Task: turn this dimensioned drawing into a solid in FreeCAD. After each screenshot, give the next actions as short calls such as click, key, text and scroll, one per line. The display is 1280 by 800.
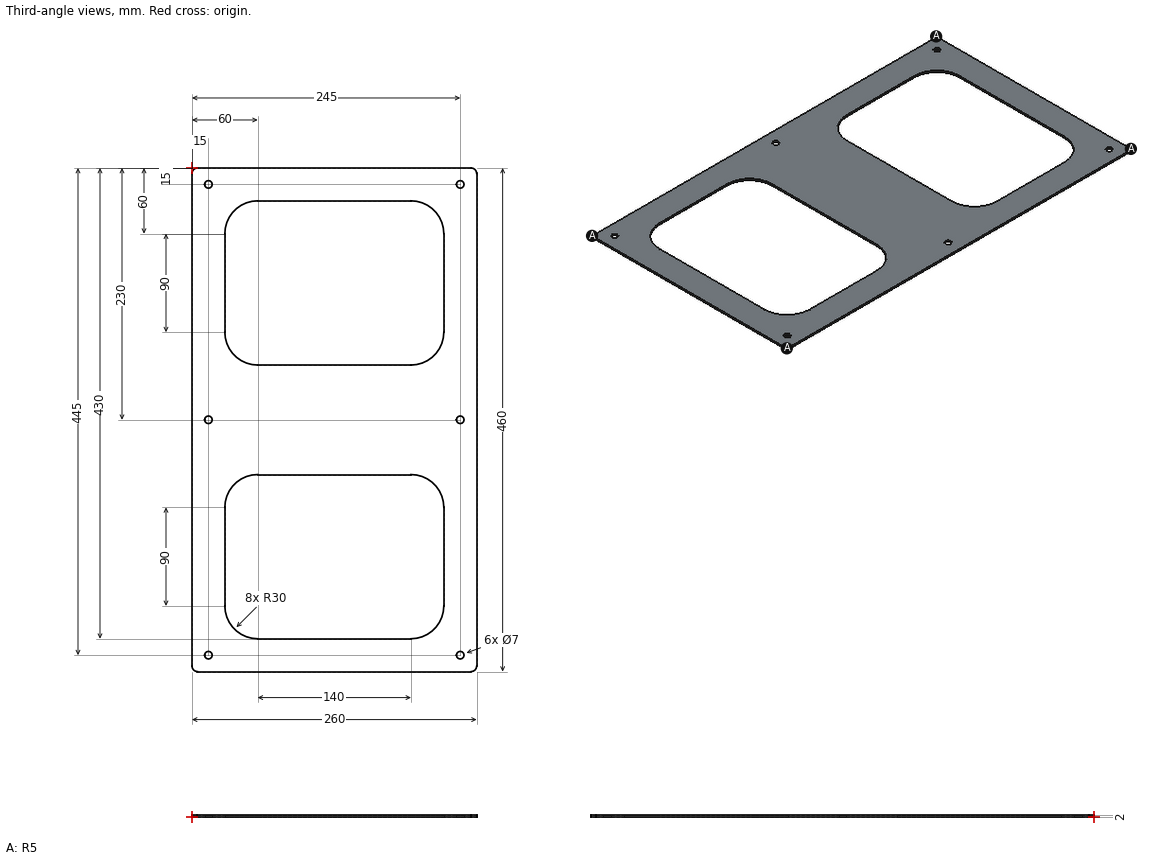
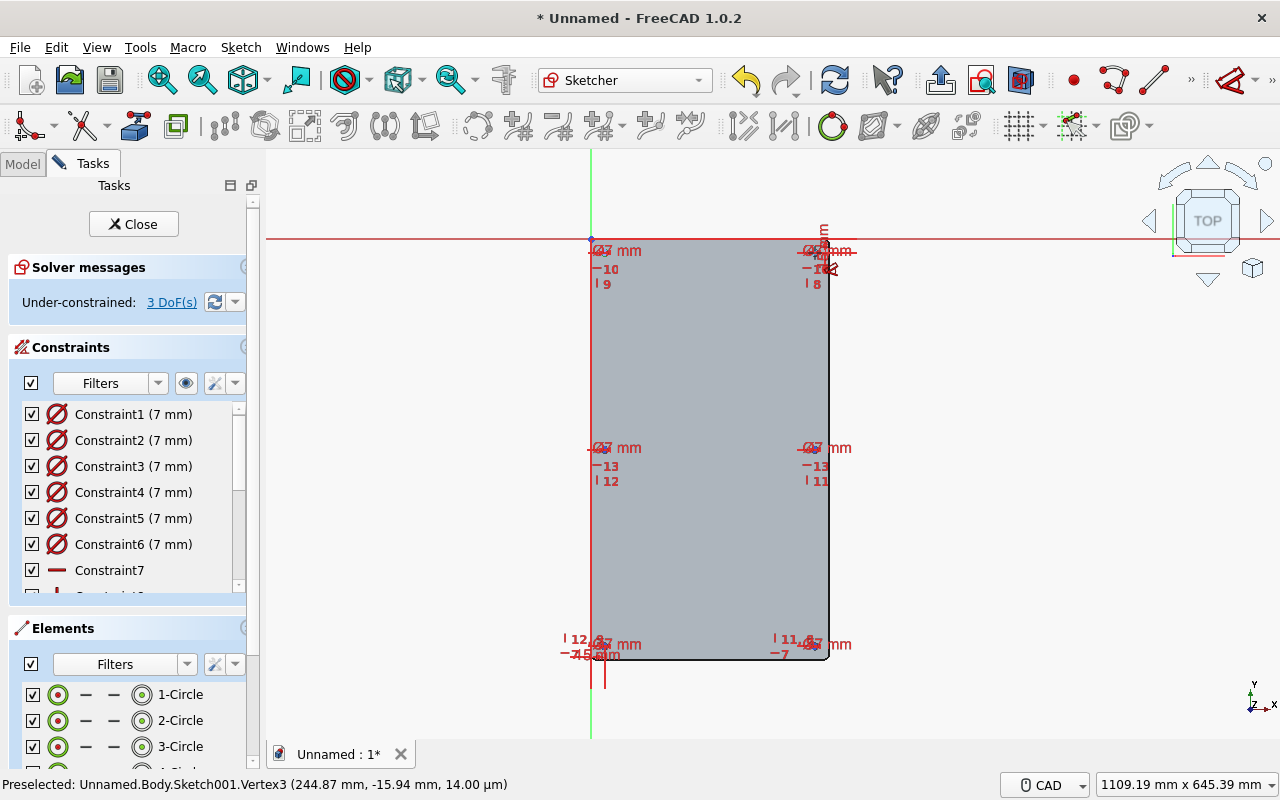
click(815, 646)
click(703, 205)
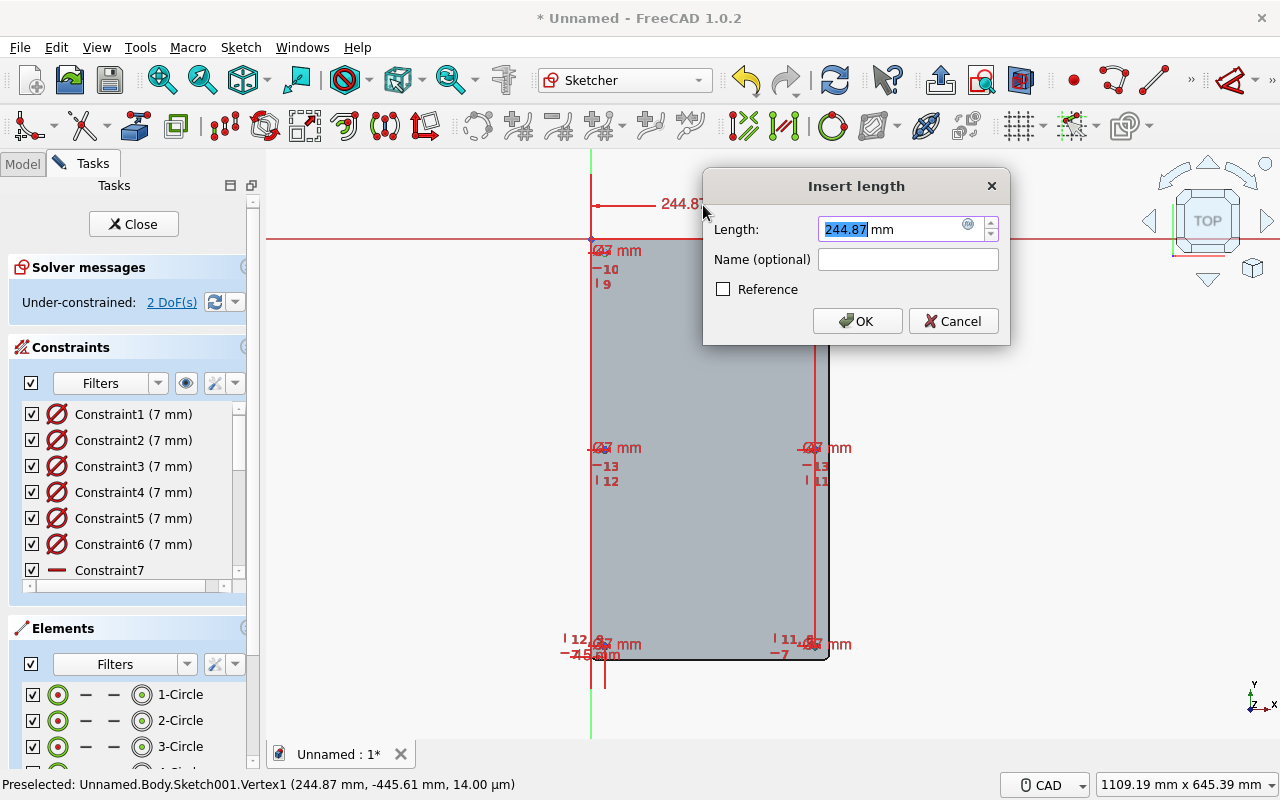
text(245)
key(Return)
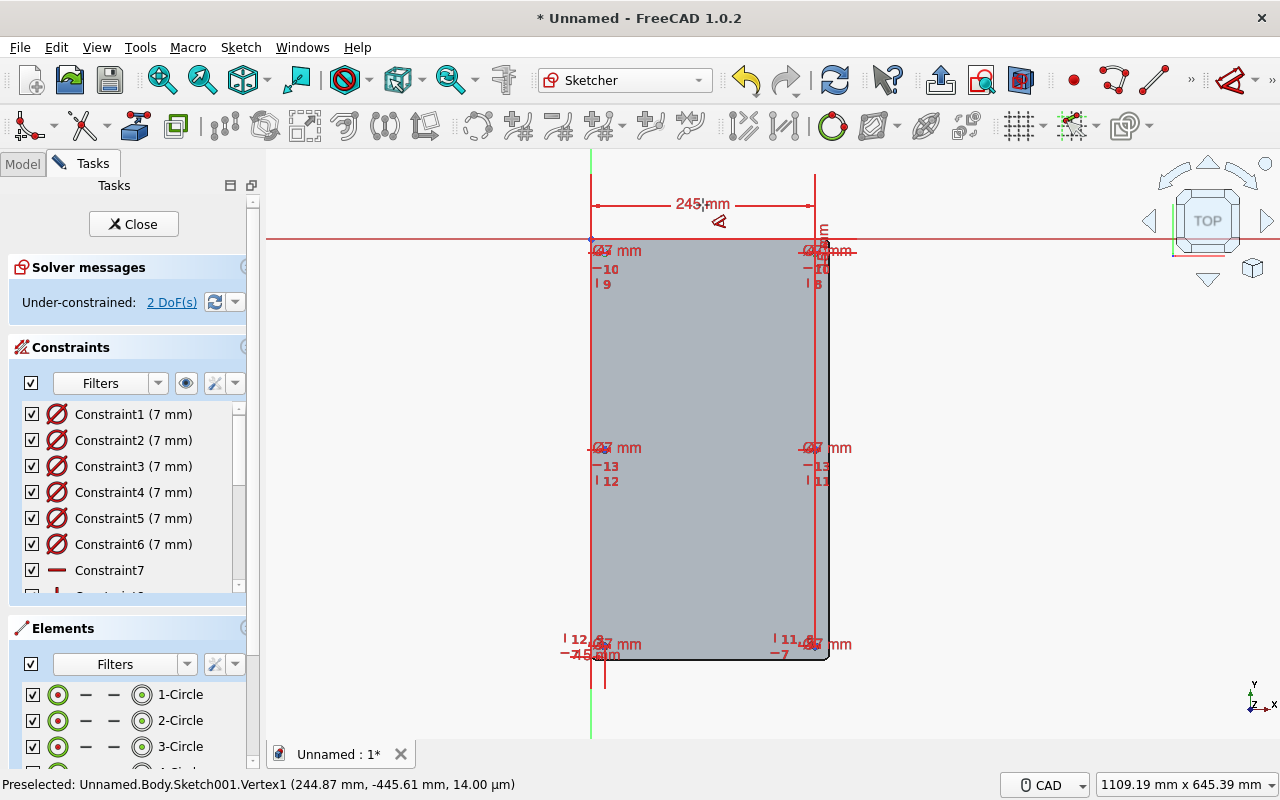
click(815, 646)
click(557, 443)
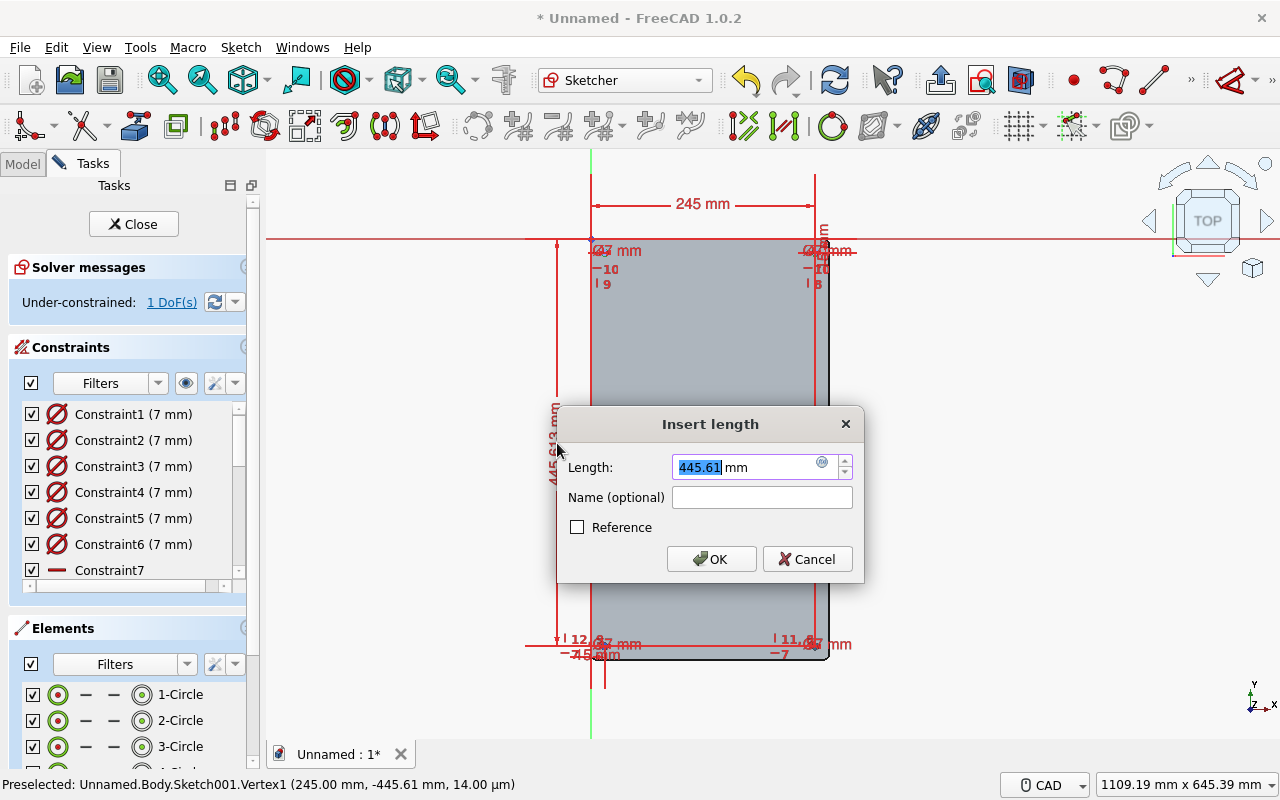
text(445)
key(Return)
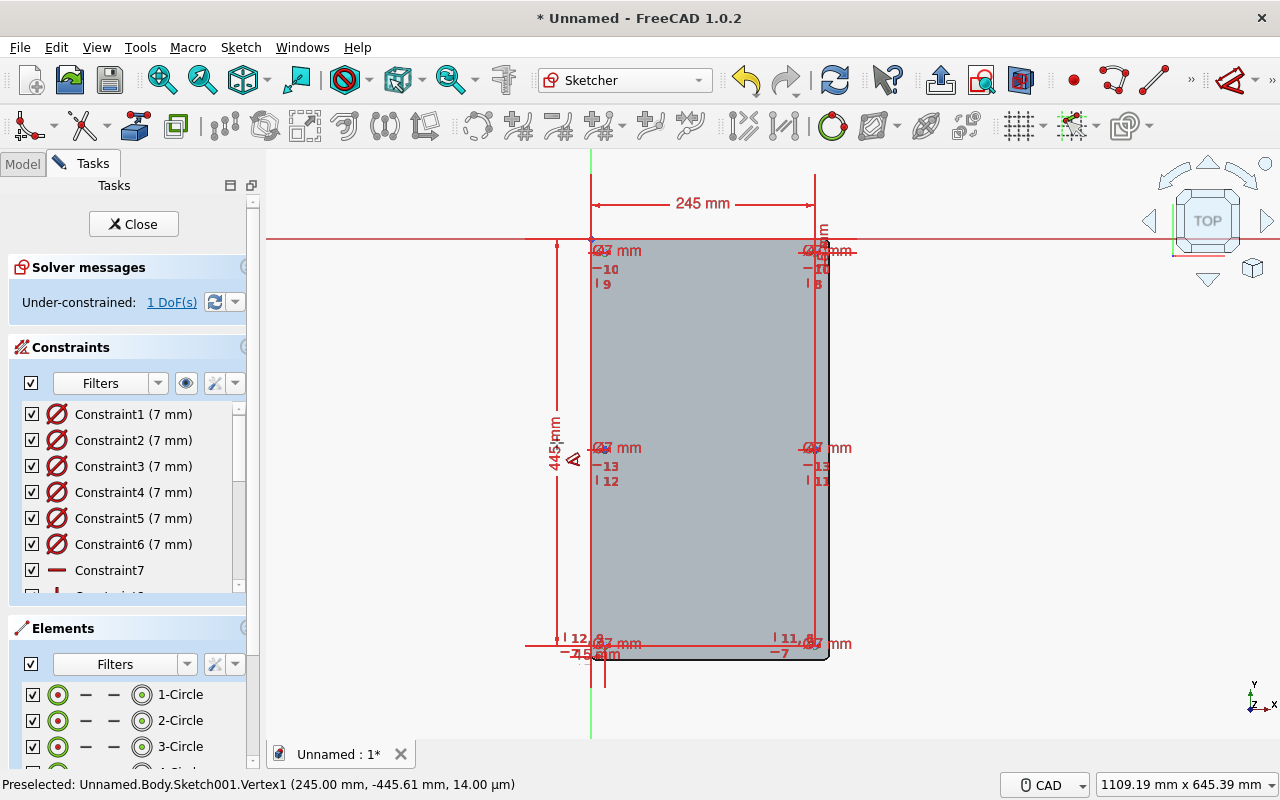
click(815, 450)
click(557, 345)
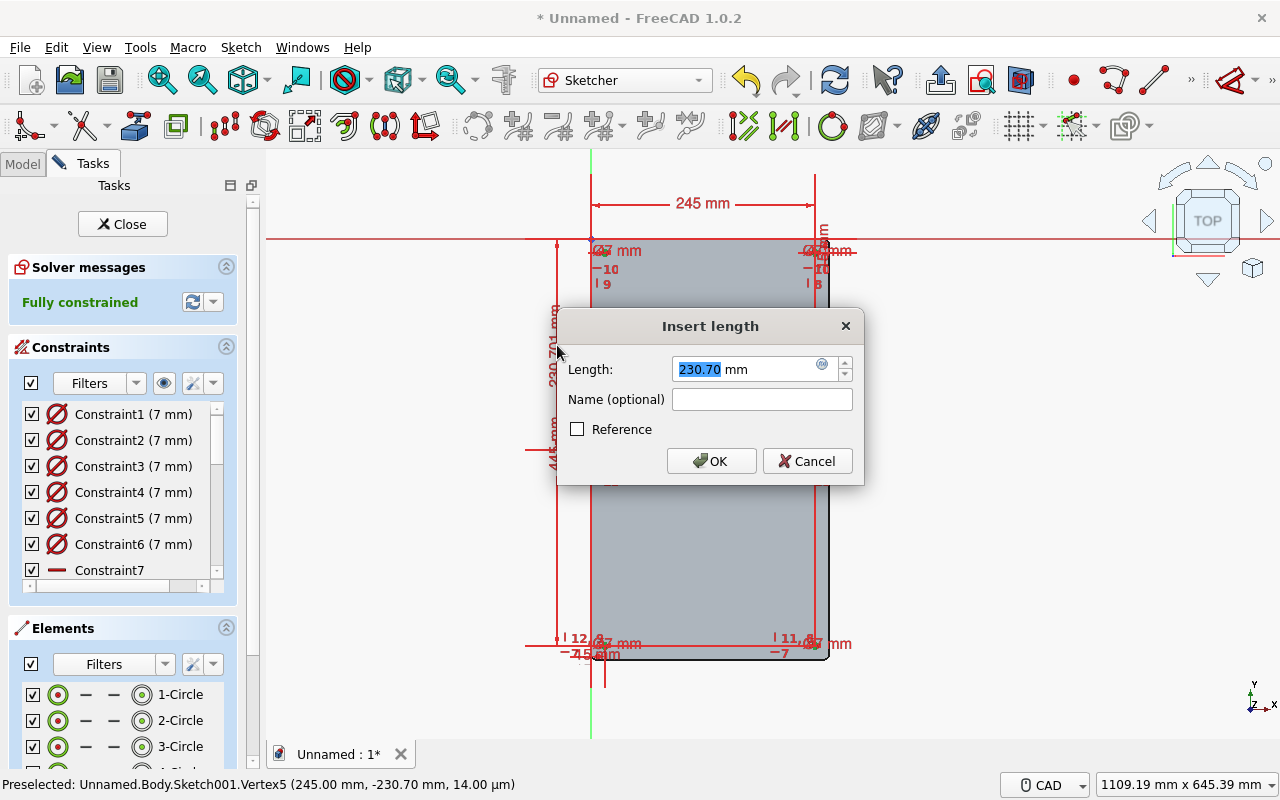
text(230)
key(Return)
key(Escape)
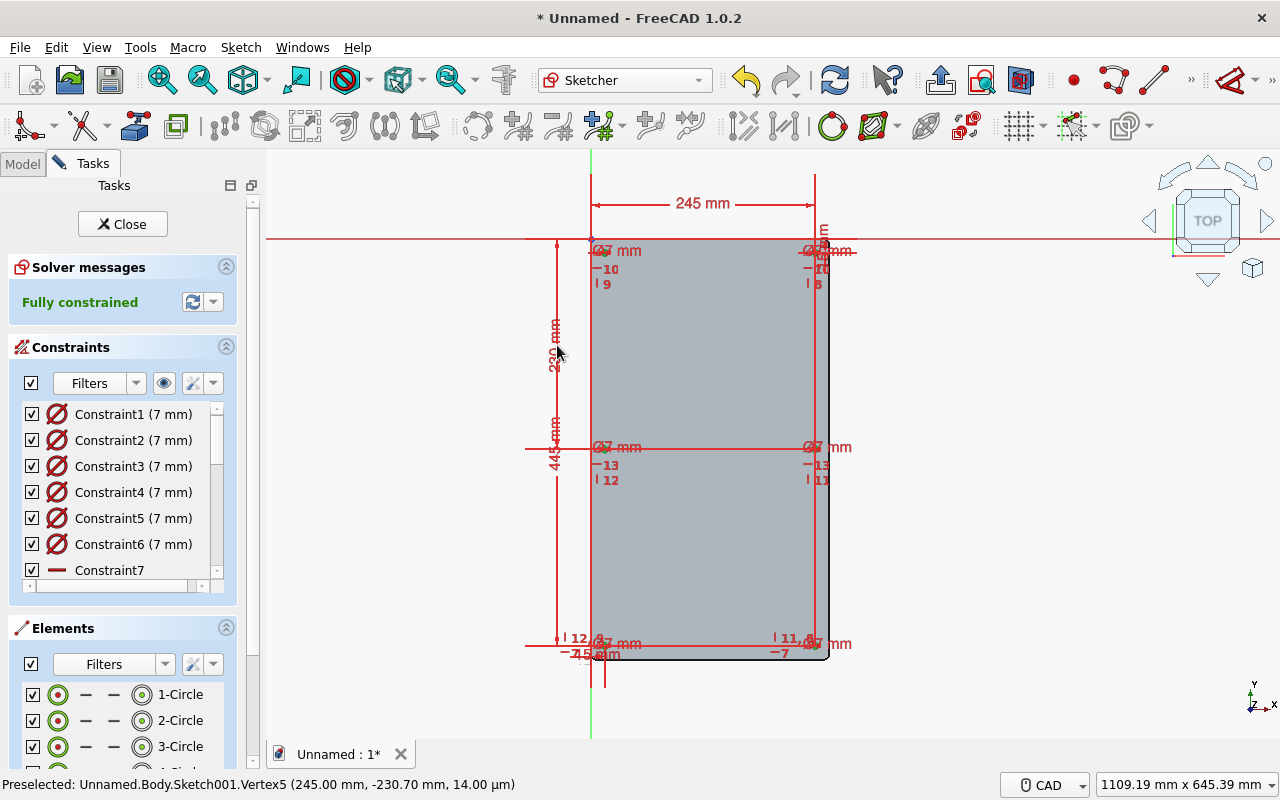
click(123, 224)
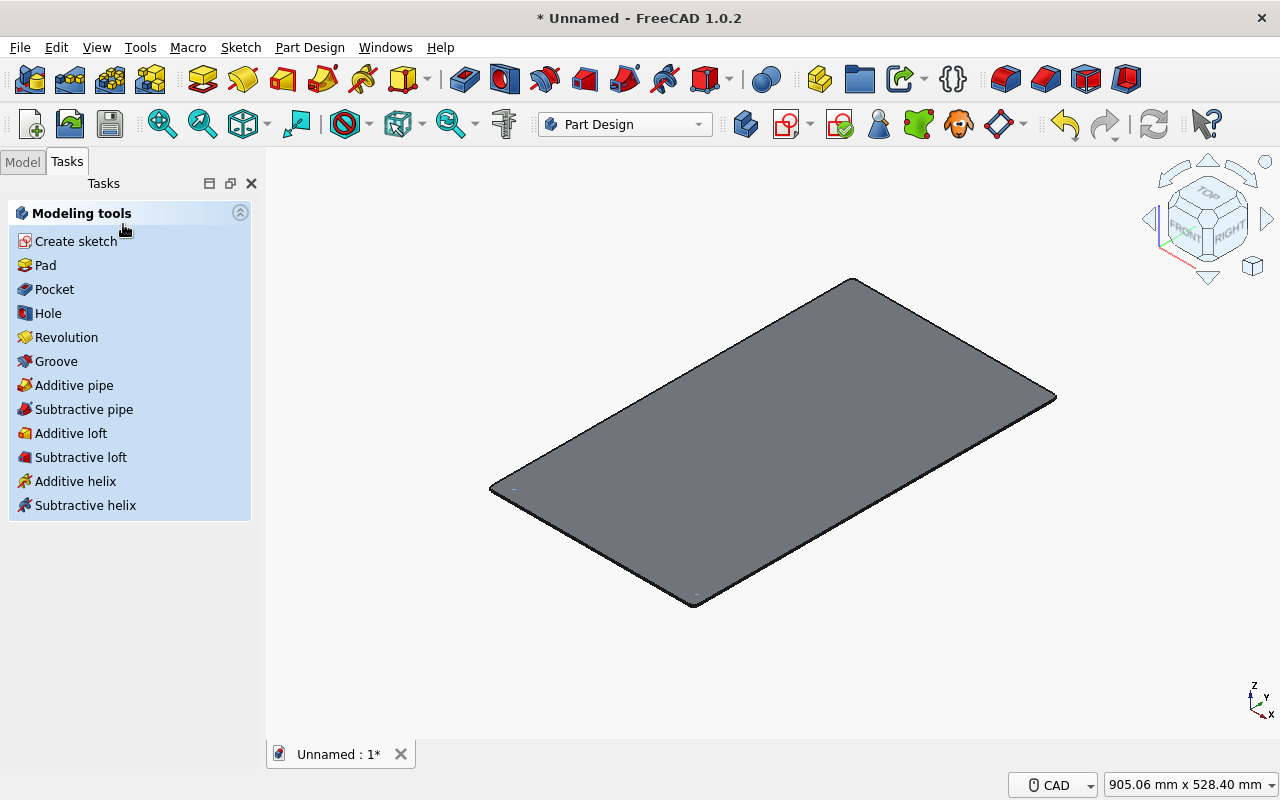
click(466, 80)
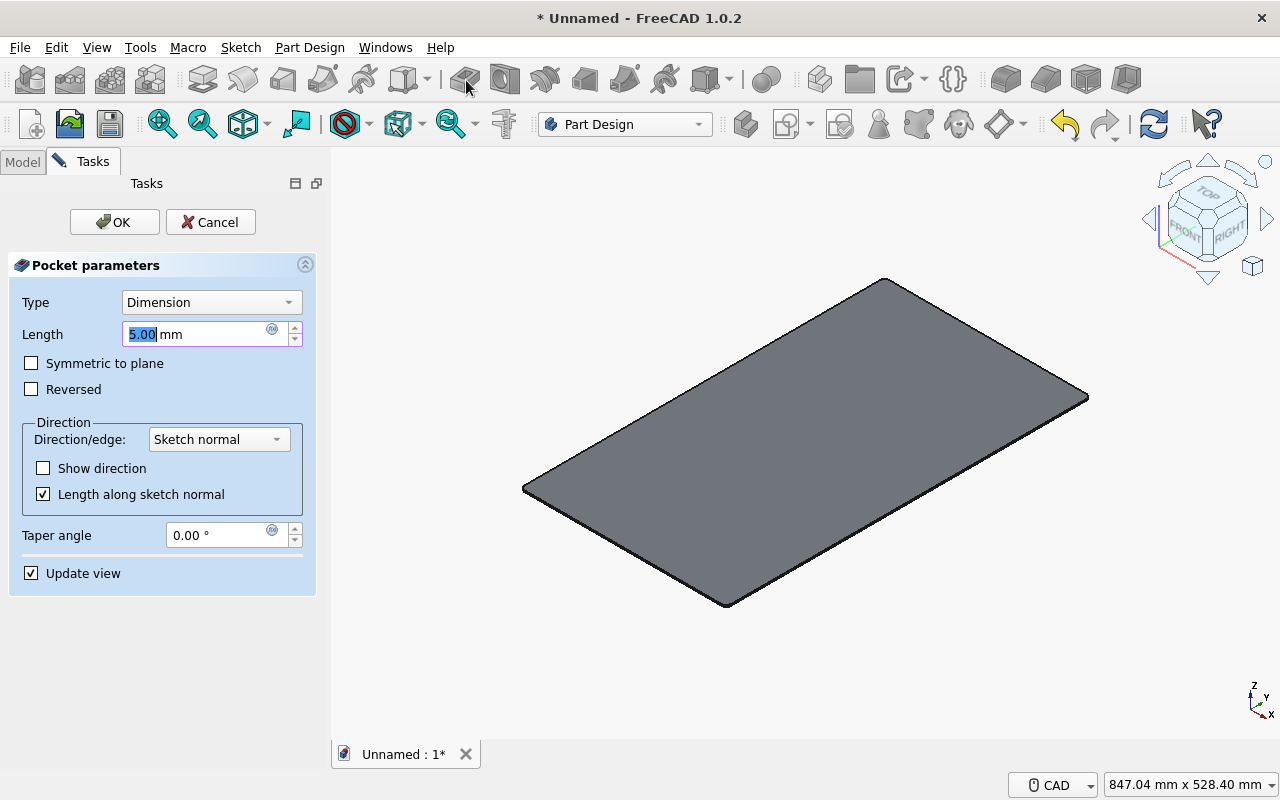
click(212, 302)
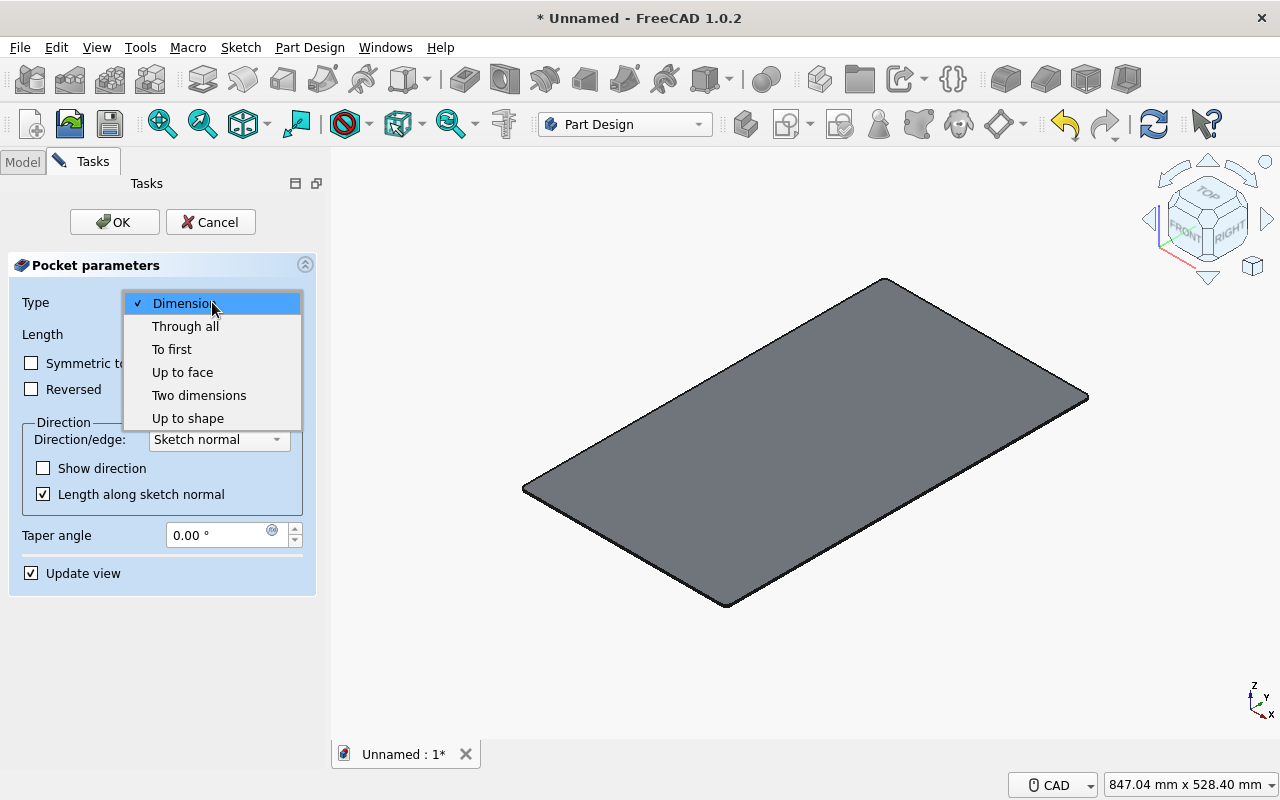
click(212, 326)